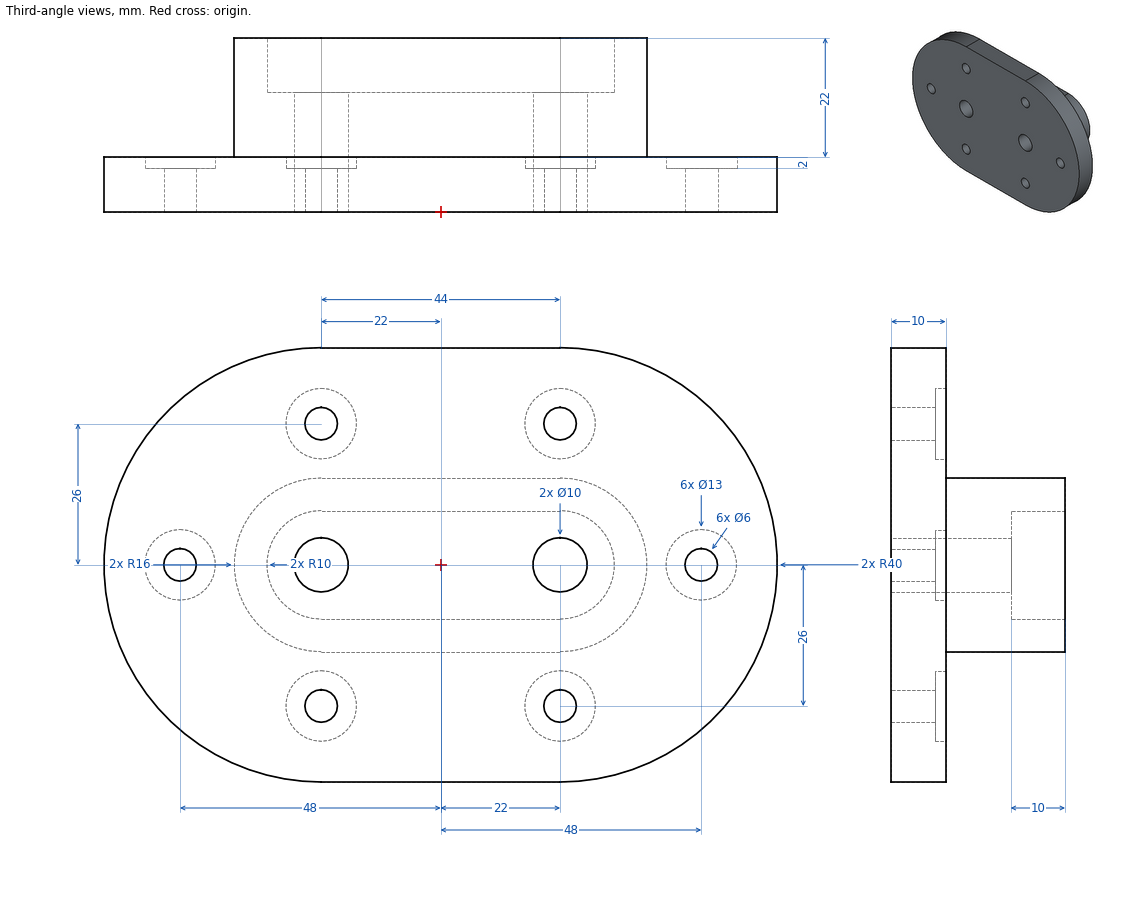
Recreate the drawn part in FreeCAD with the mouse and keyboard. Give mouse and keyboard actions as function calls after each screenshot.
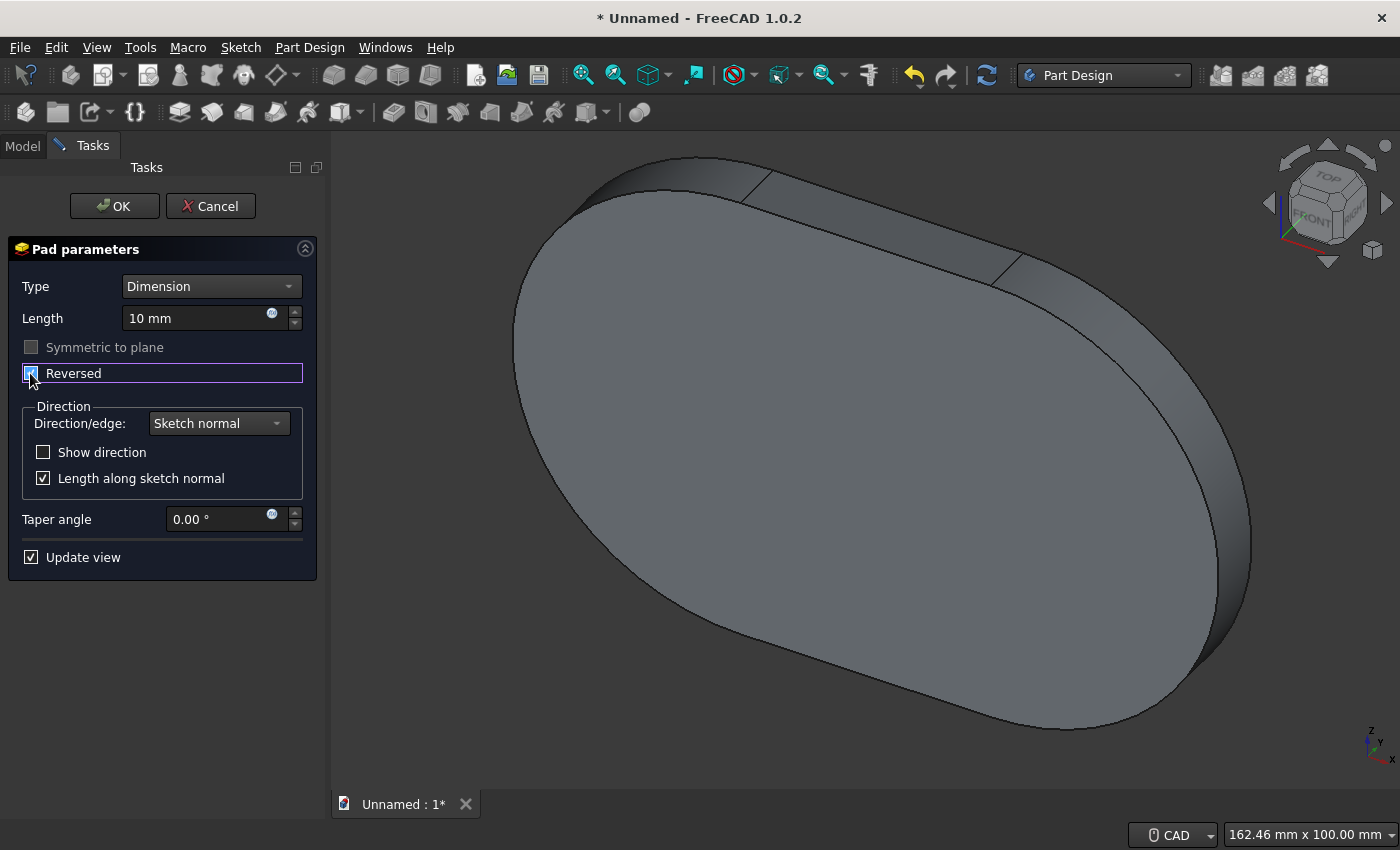
click(115, 206)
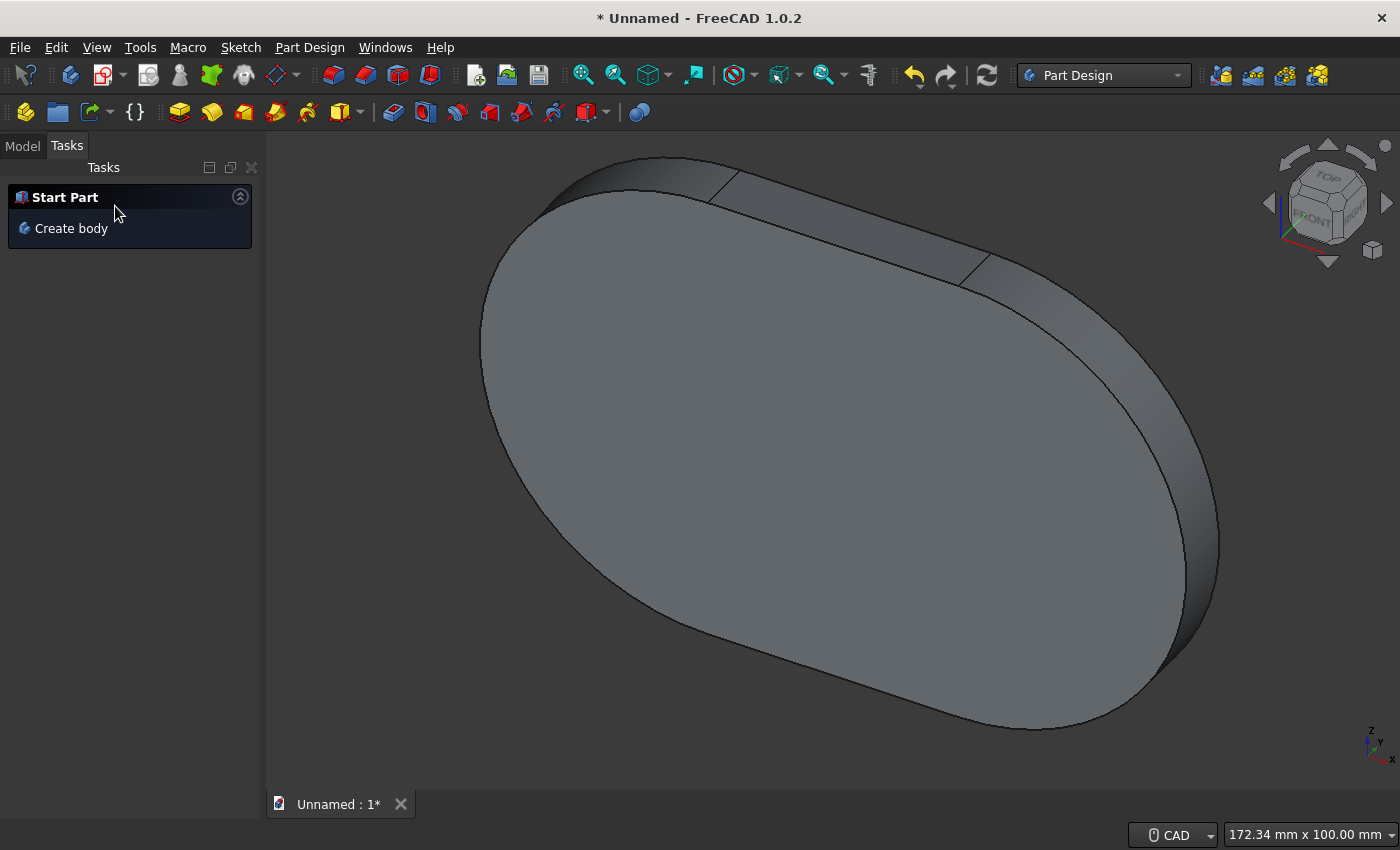
click(584, 76)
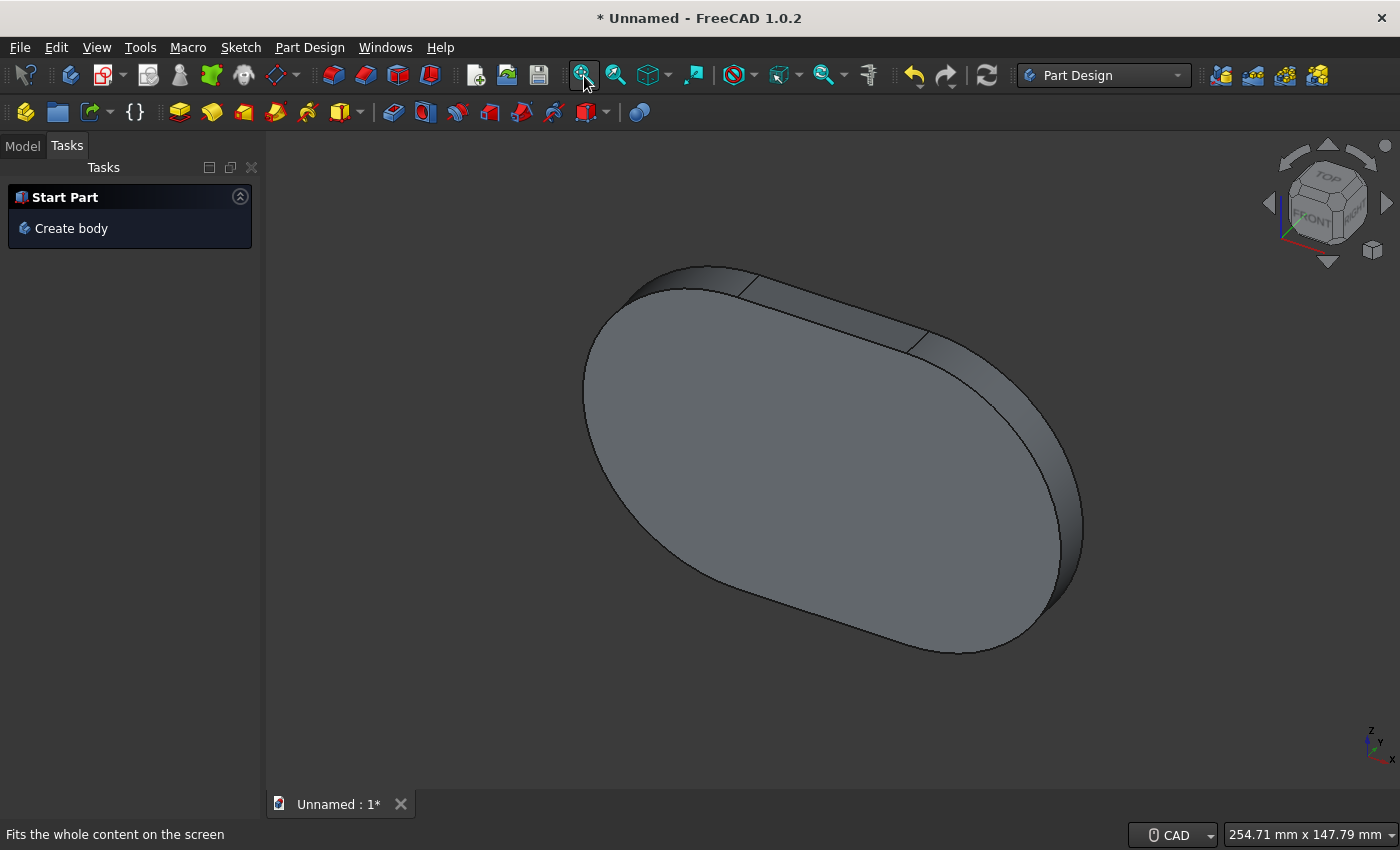
key(4)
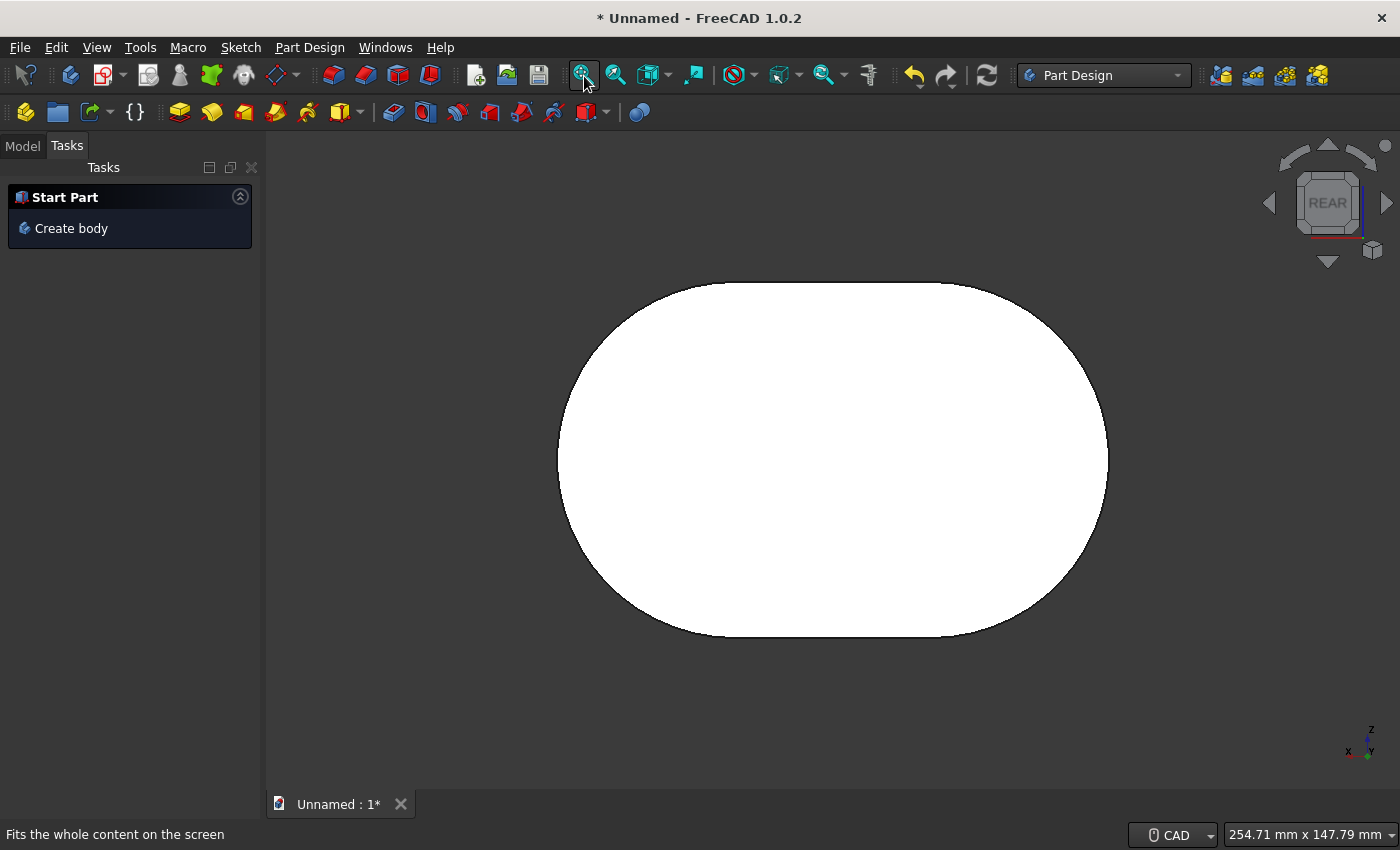
click(754, 459)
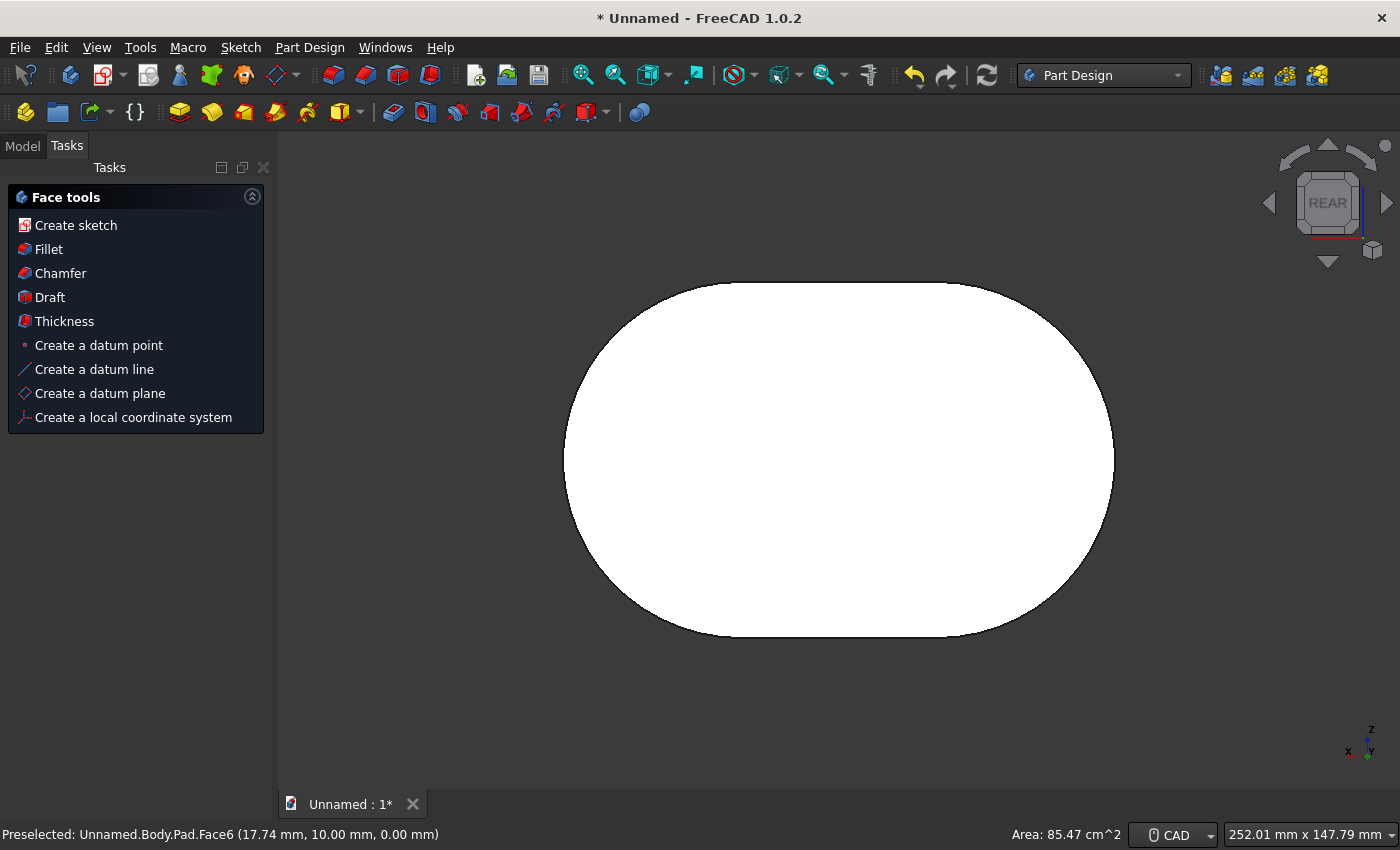
click(104, 76)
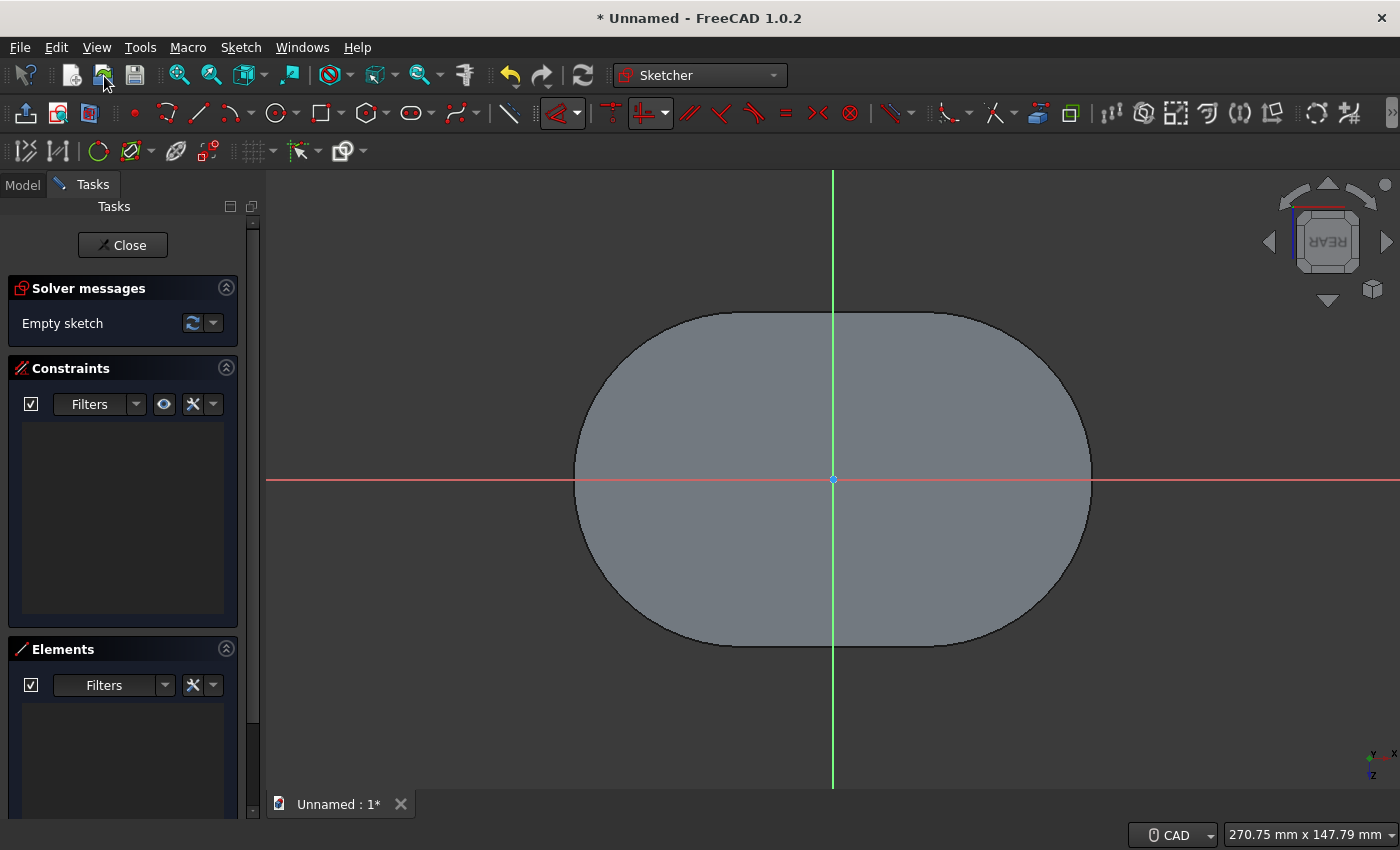
scroll(889, 480, up, 4)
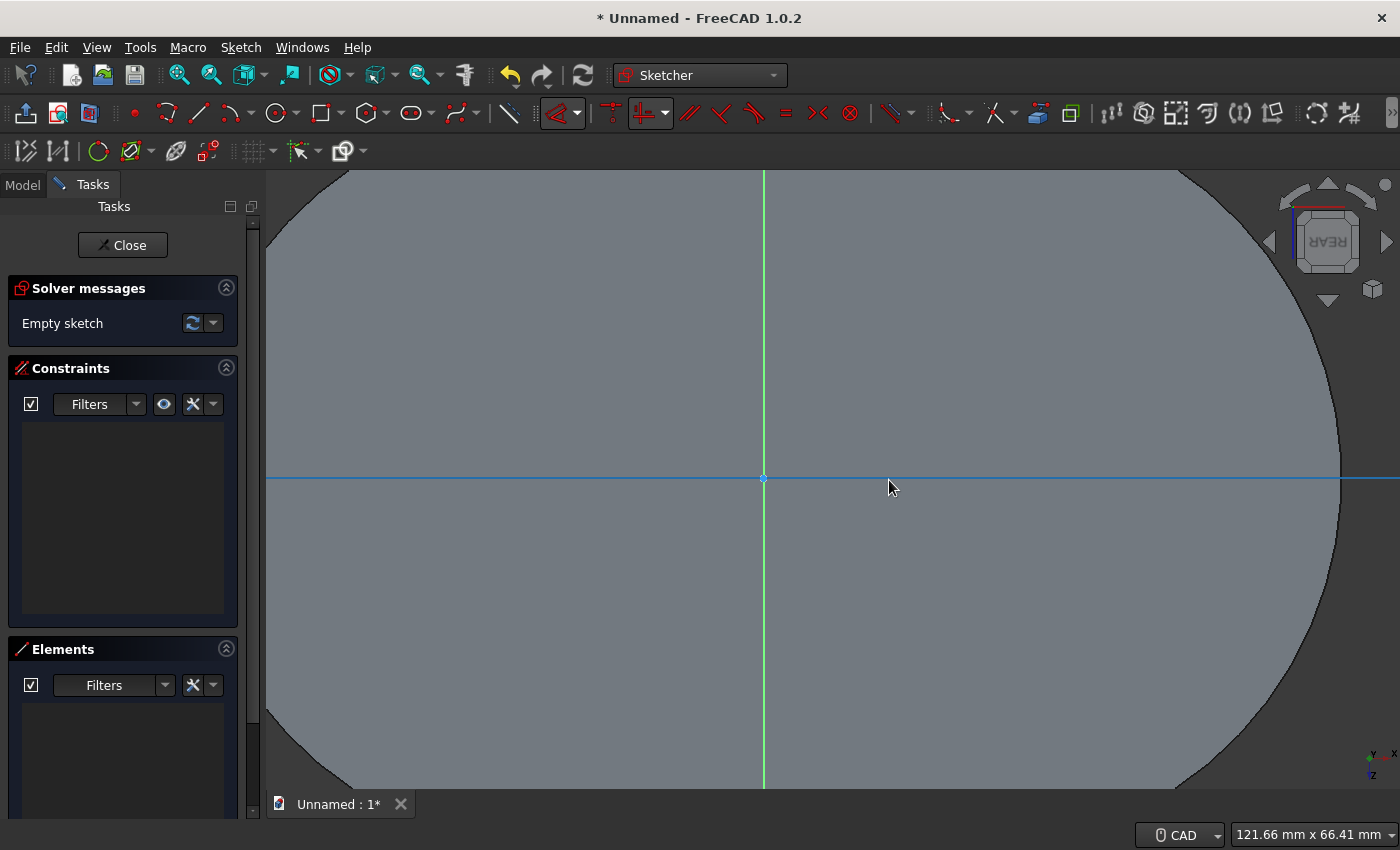
key(g)
key(s)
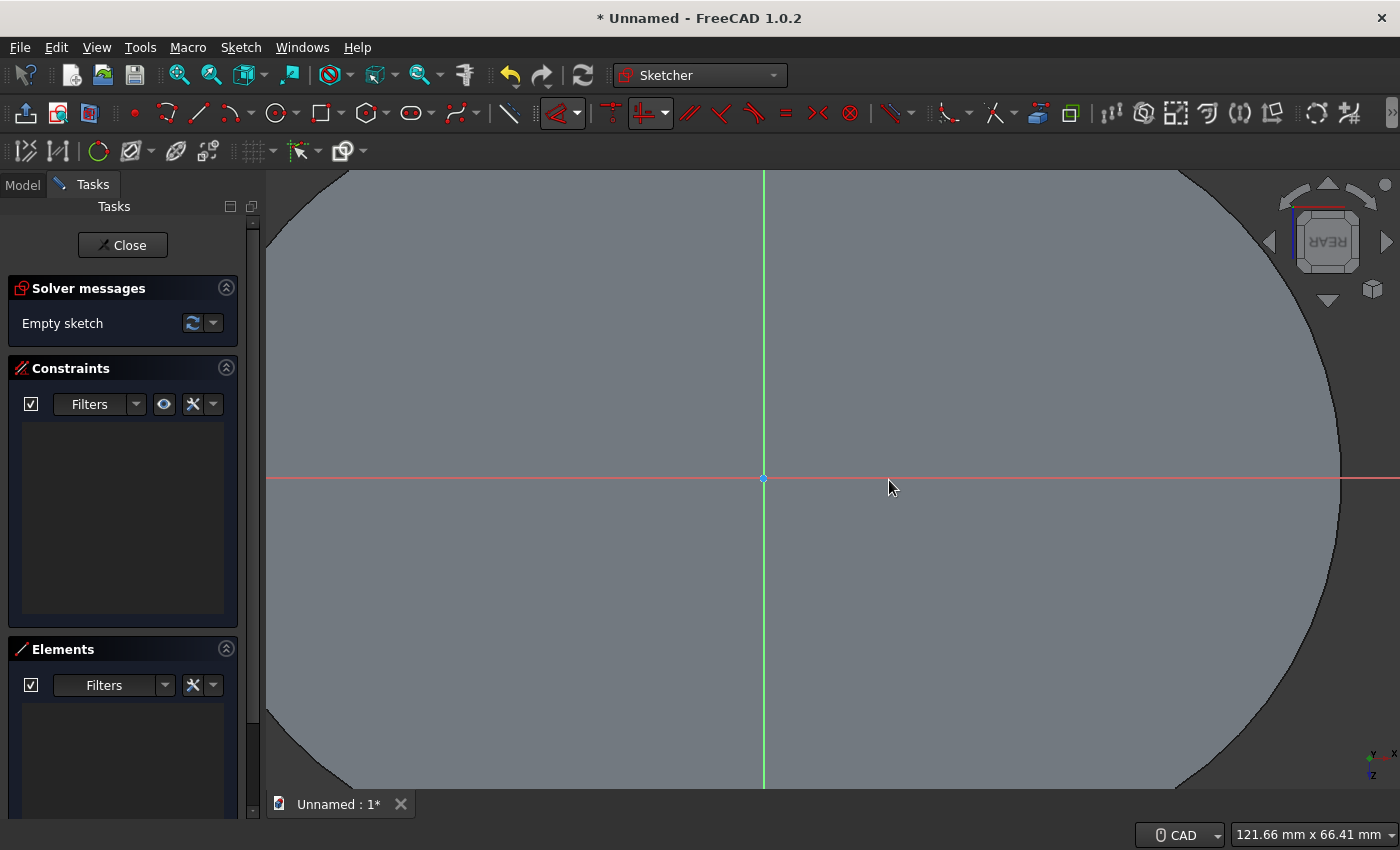
click(559, 478)